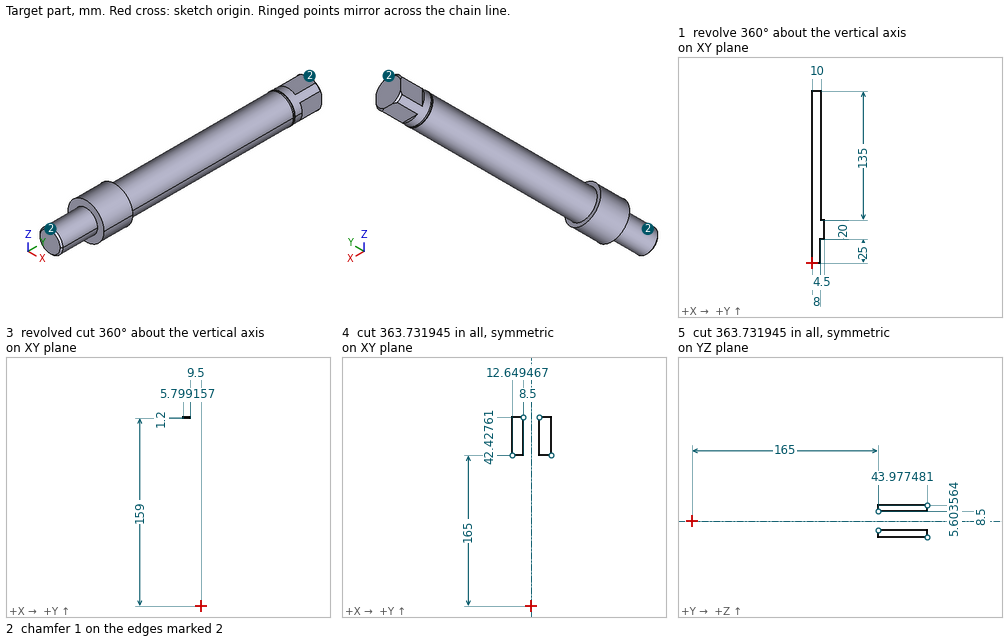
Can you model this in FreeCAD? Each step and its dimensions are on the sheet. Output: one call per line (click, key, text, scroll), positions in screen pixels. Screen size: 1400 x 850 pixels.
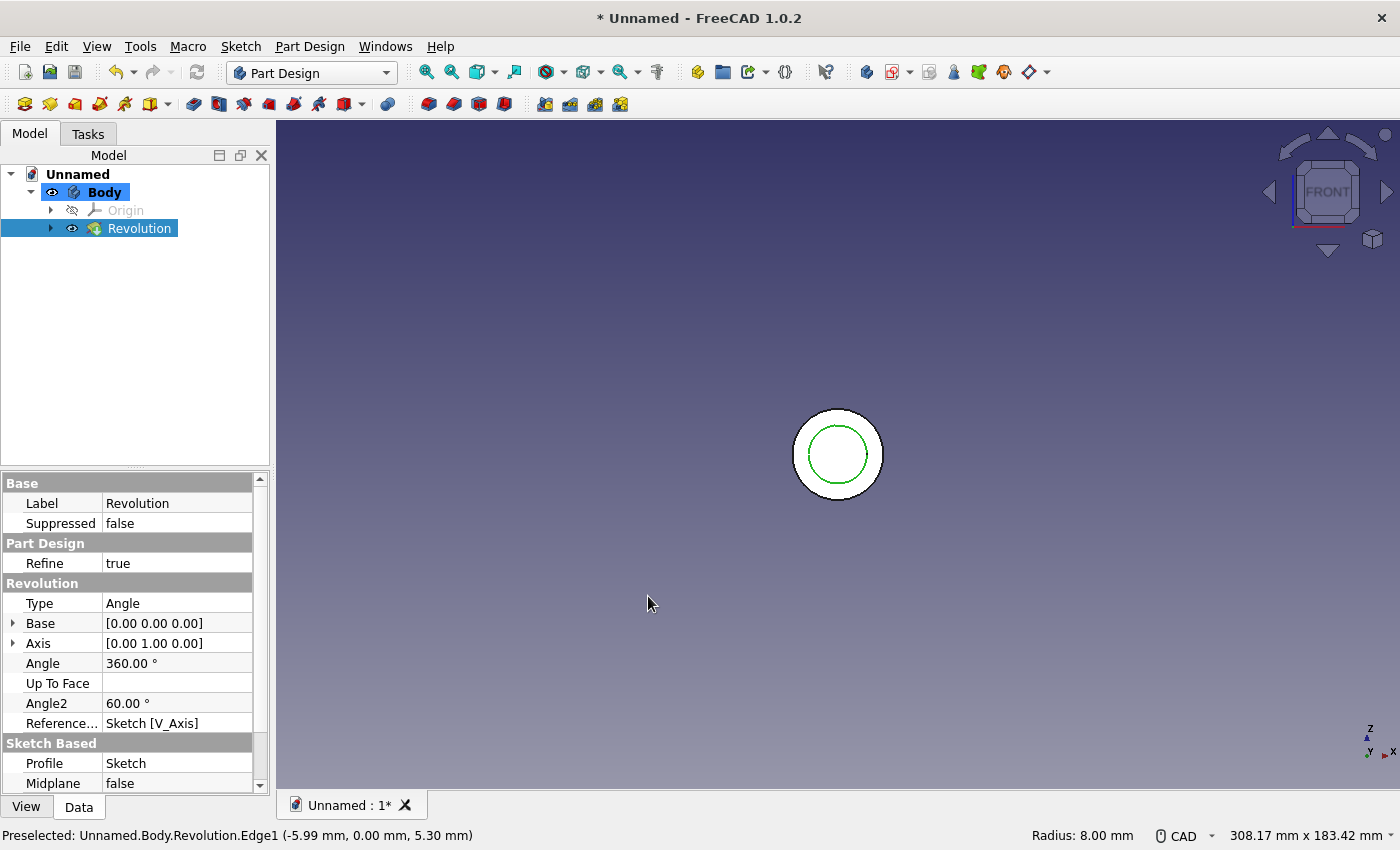
click(427, 72)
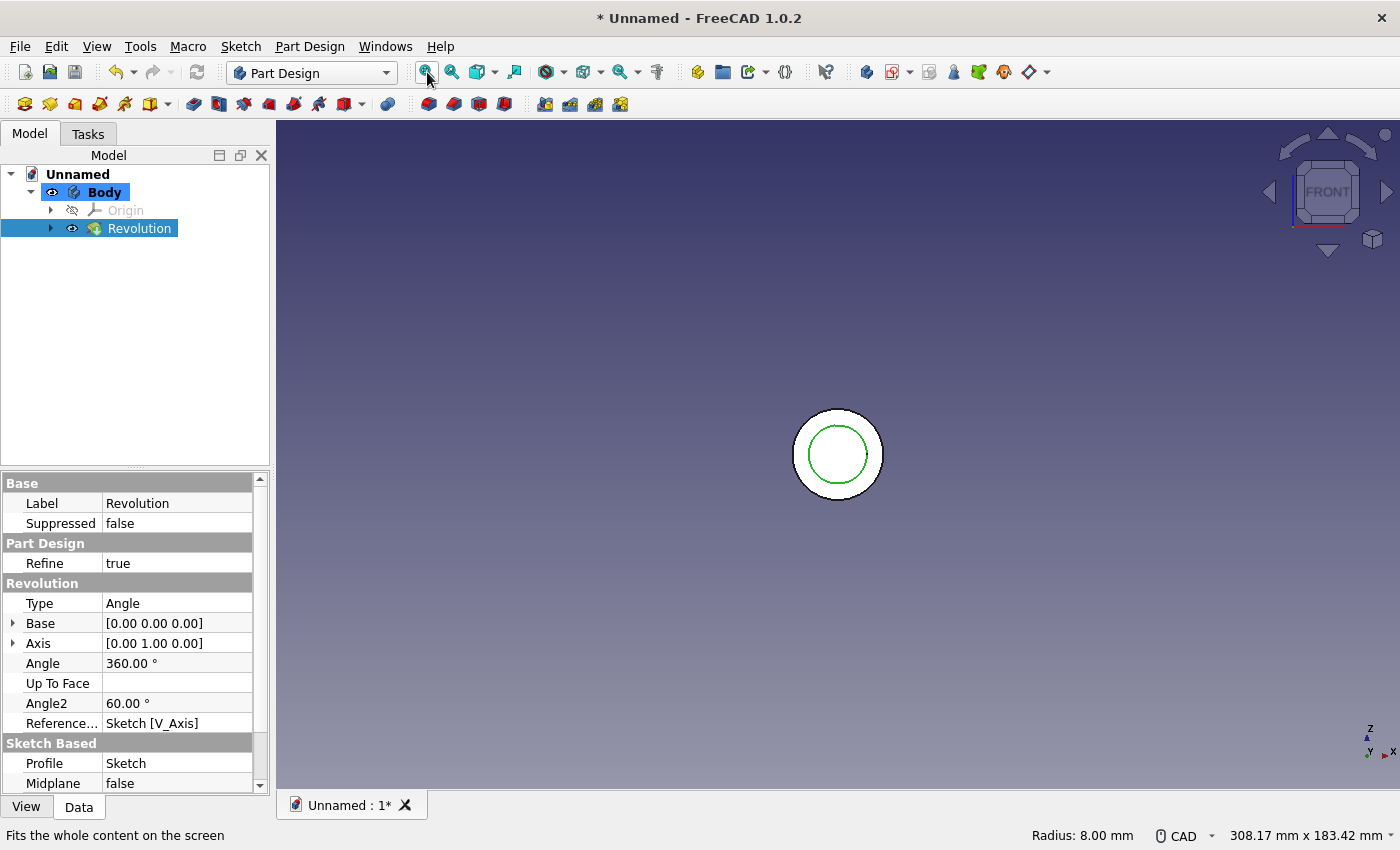
key(3)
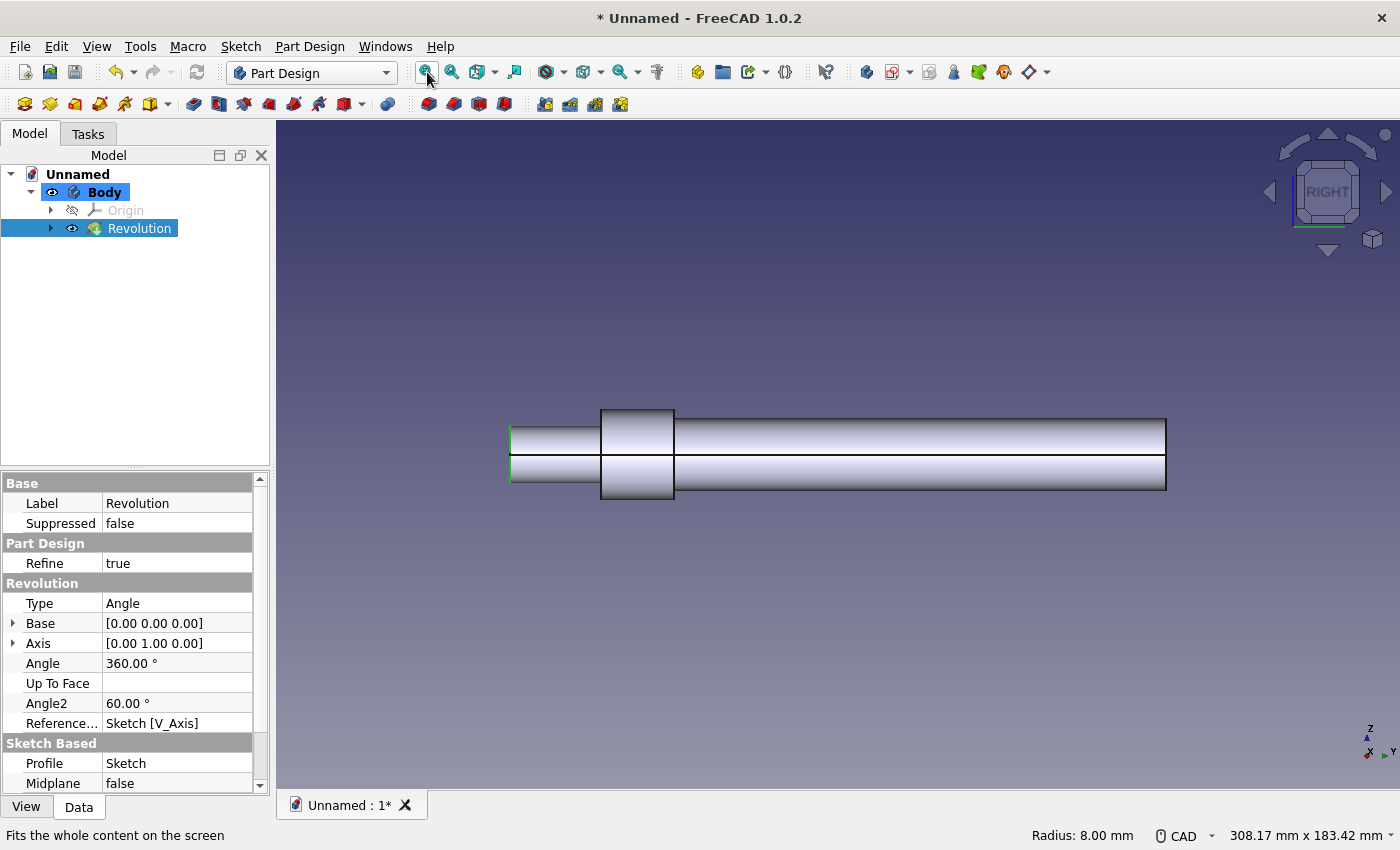
click(1166, 432, ctrl)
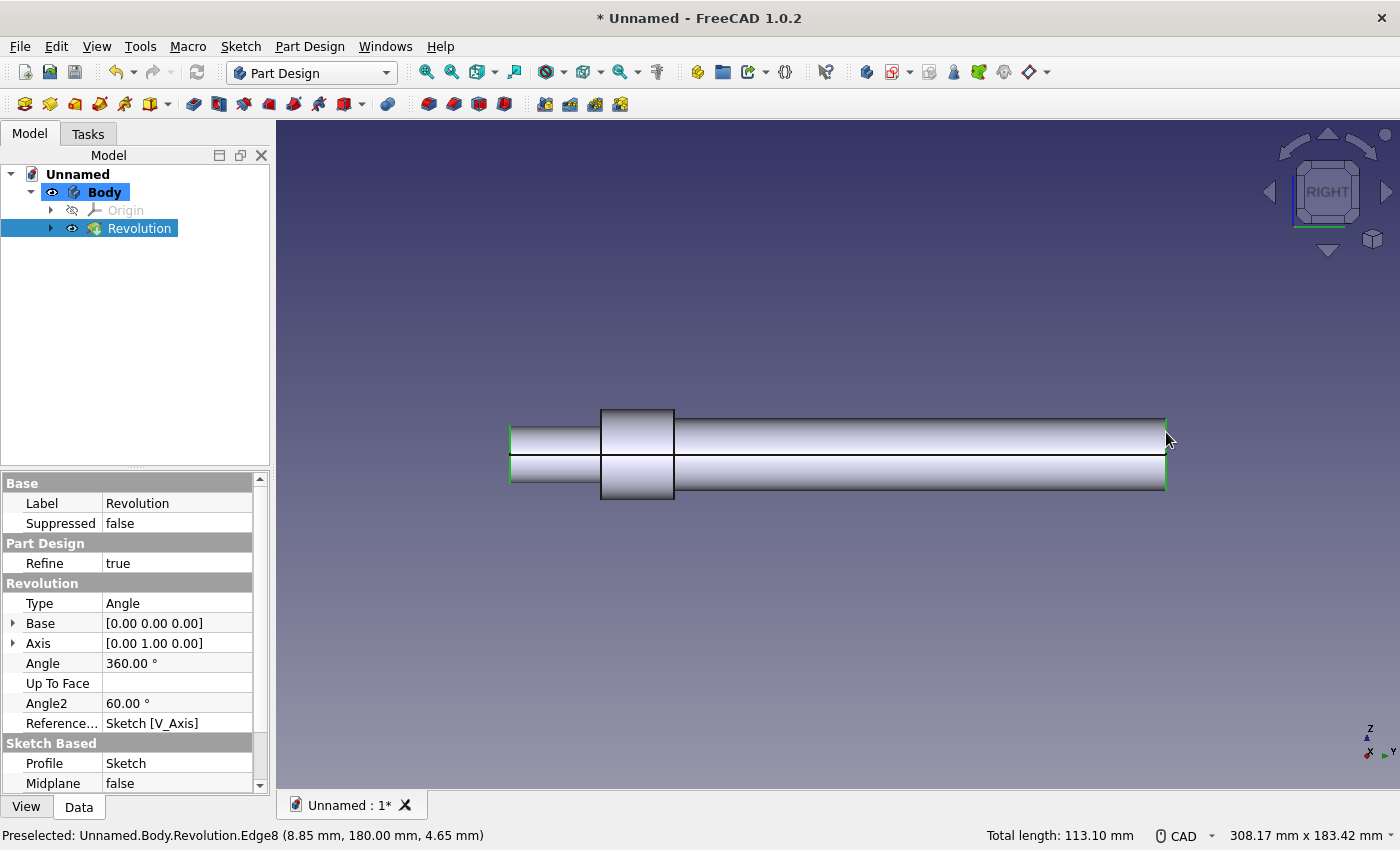
click(454, 104)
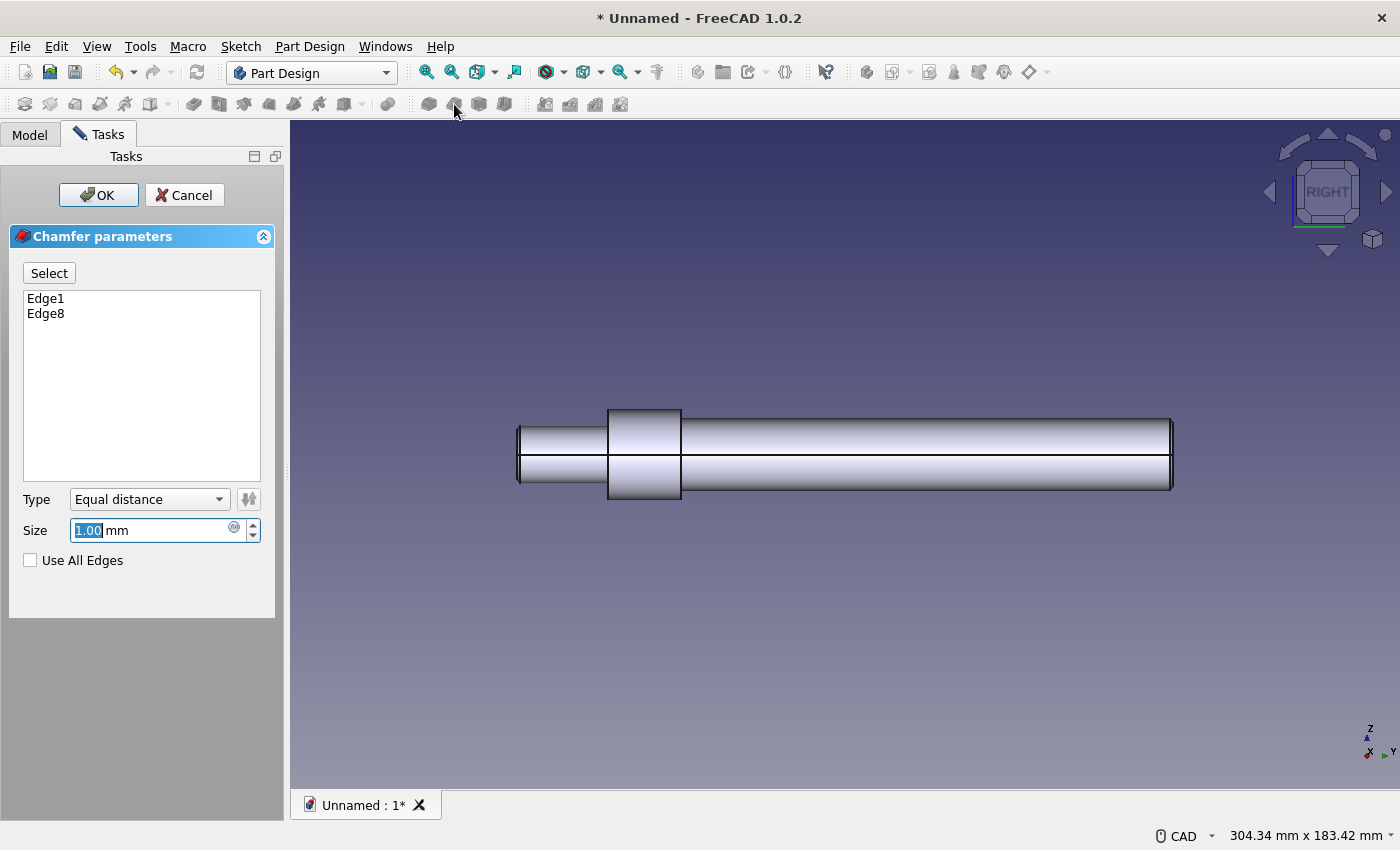
text(1)
key(Tab)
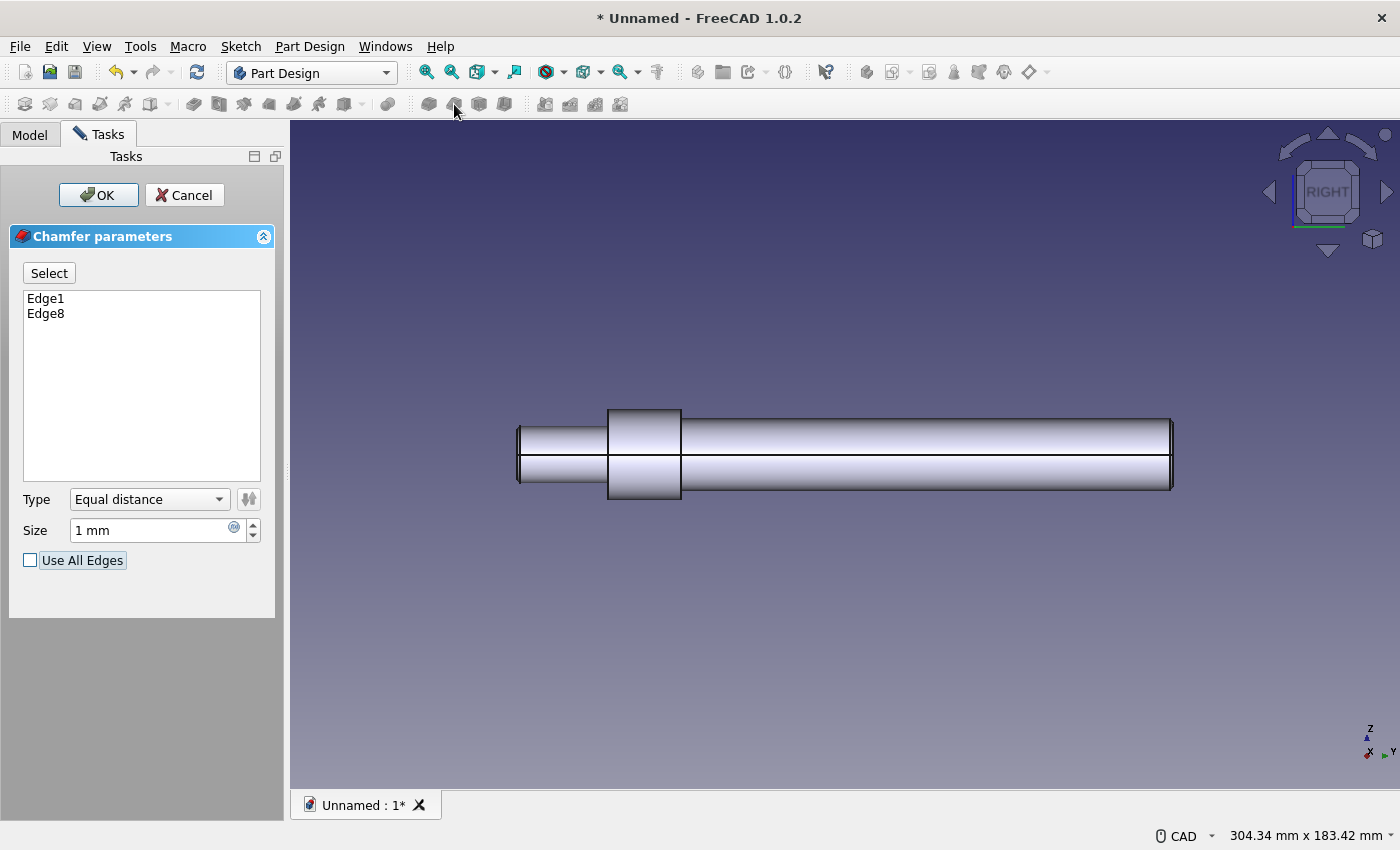
click(99, 195)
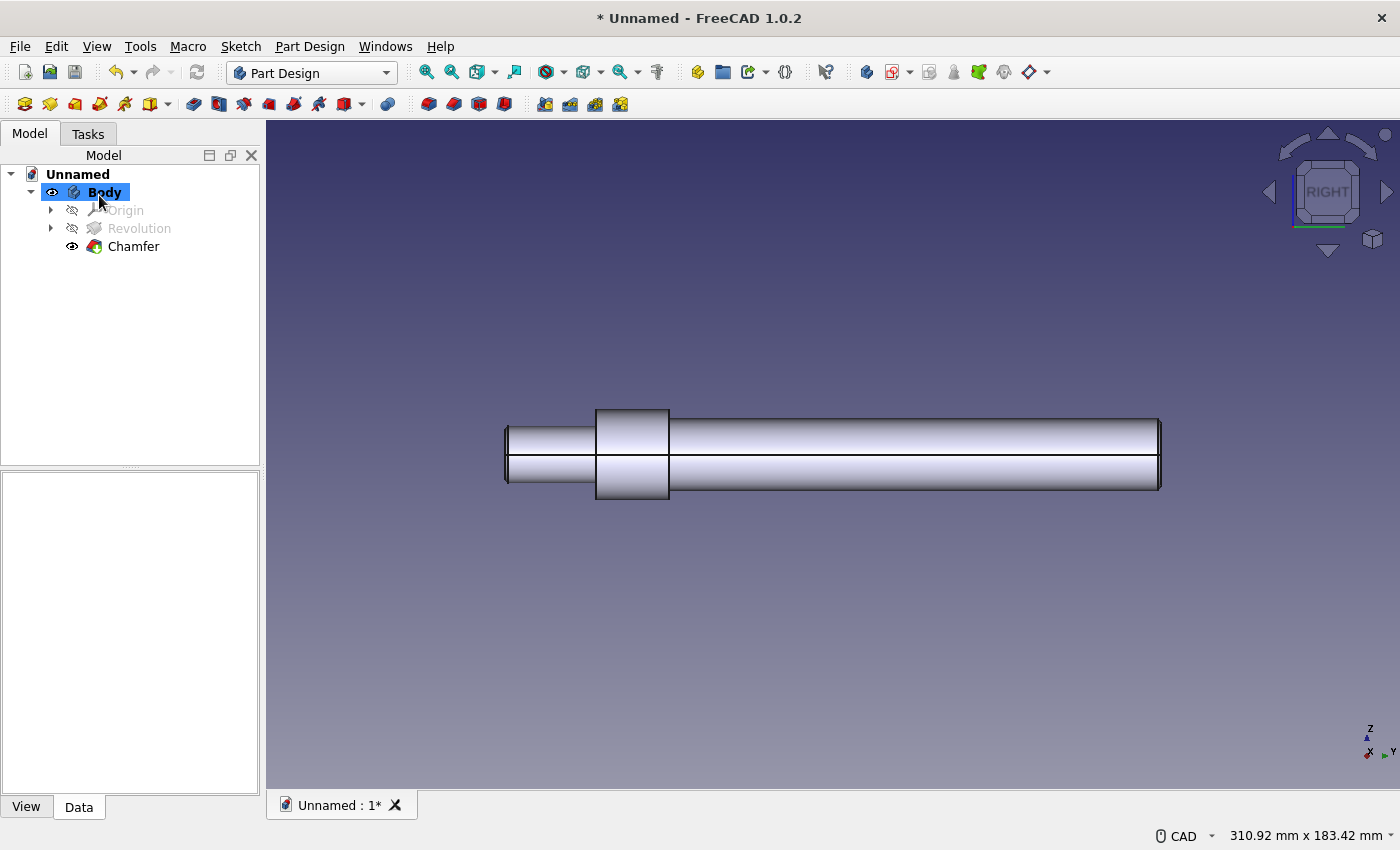
click(892, 72)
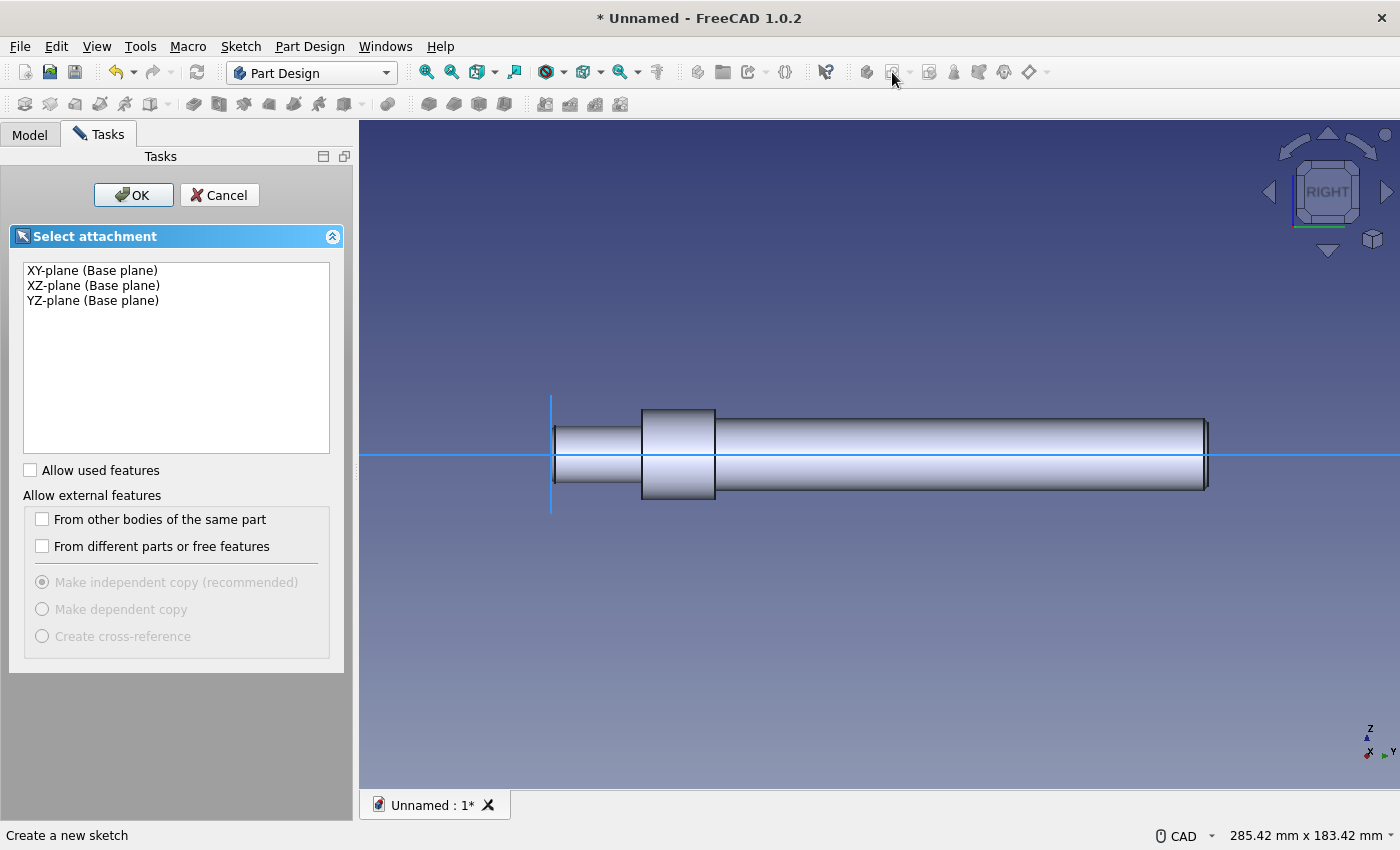
click(84, 270)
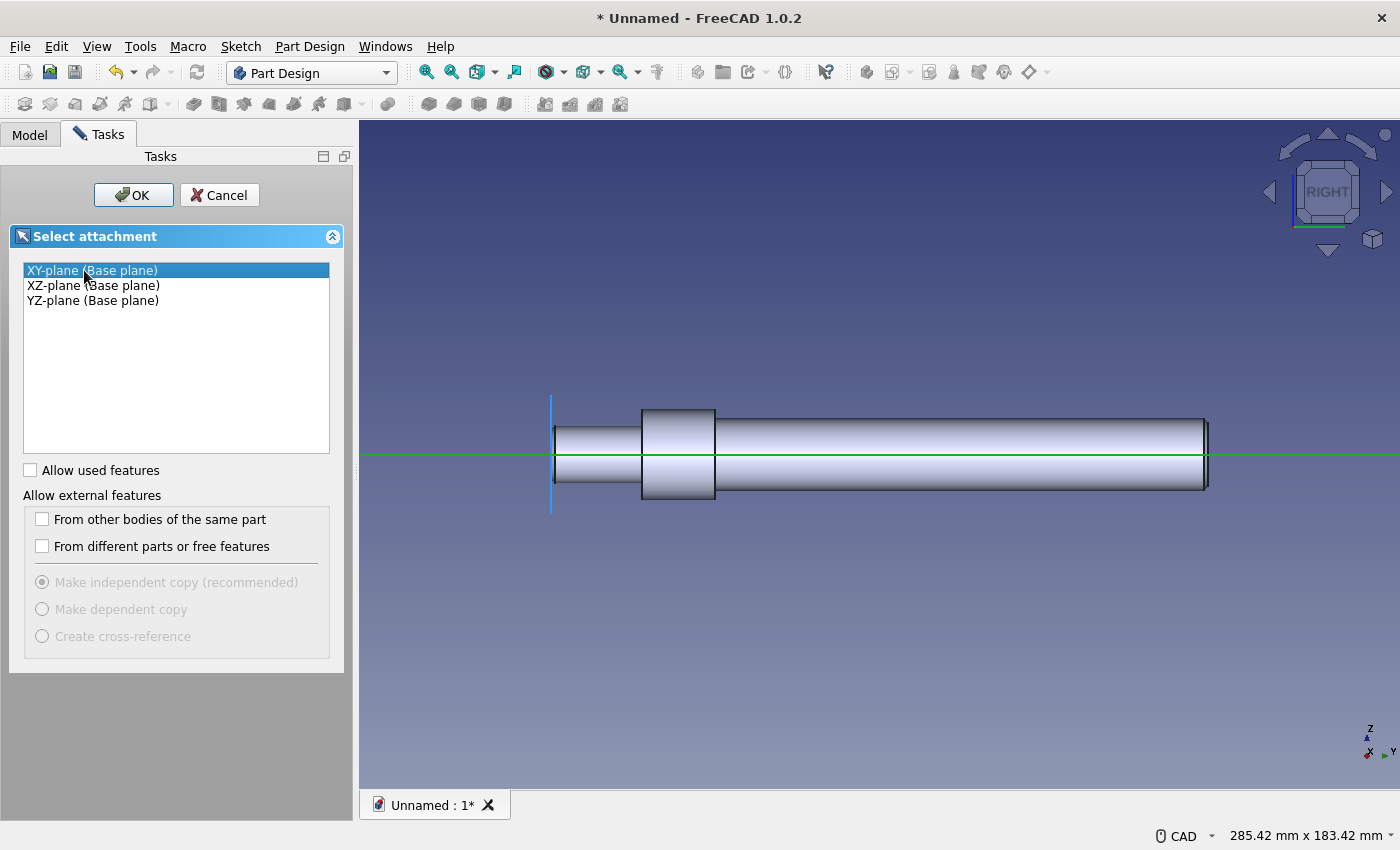
click(134, 195)